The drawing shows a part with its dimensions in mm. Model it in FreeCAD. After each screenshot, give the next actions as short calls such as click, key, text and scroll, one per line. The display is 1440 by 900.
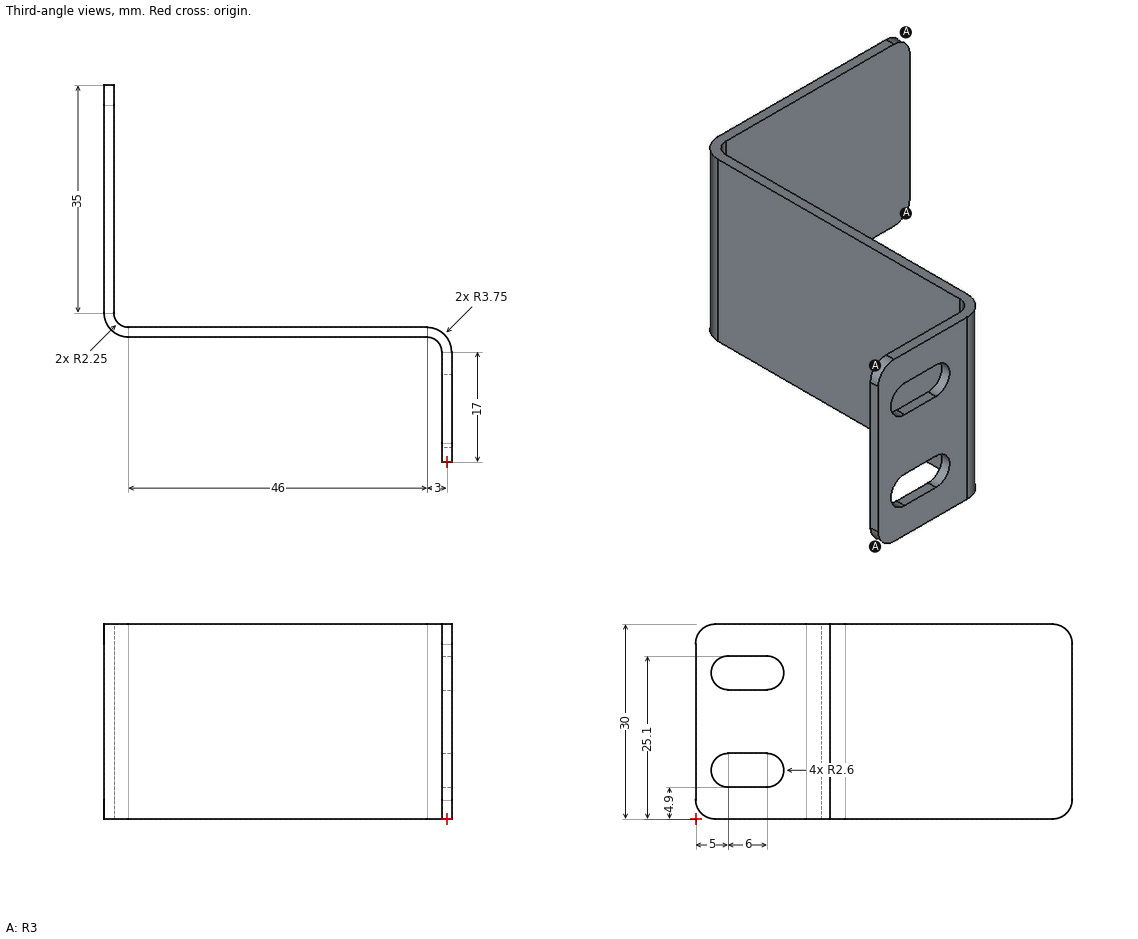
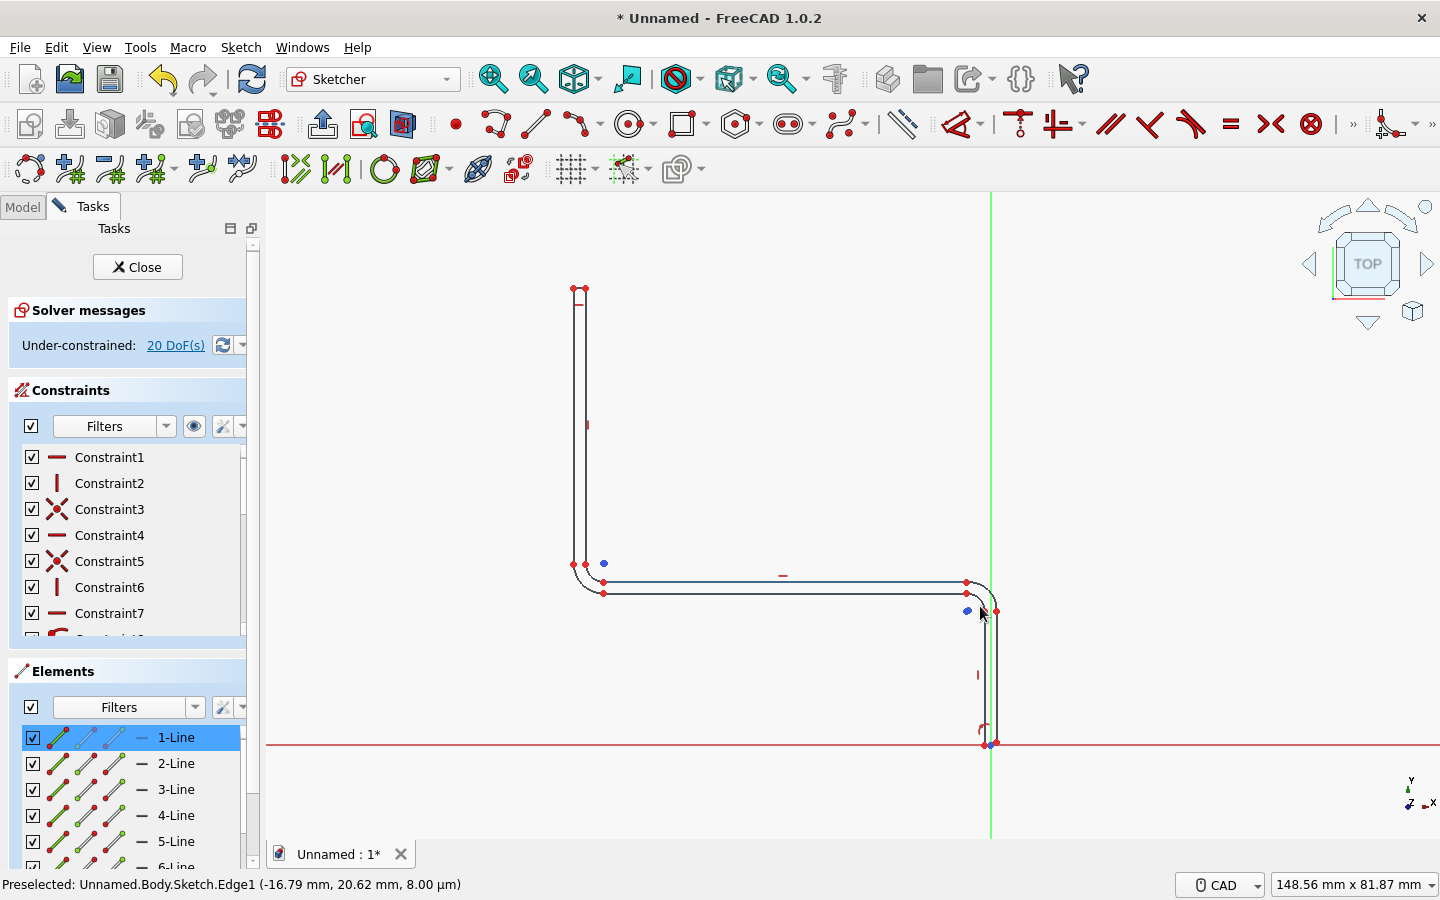
scroll(588, 572, up, 3)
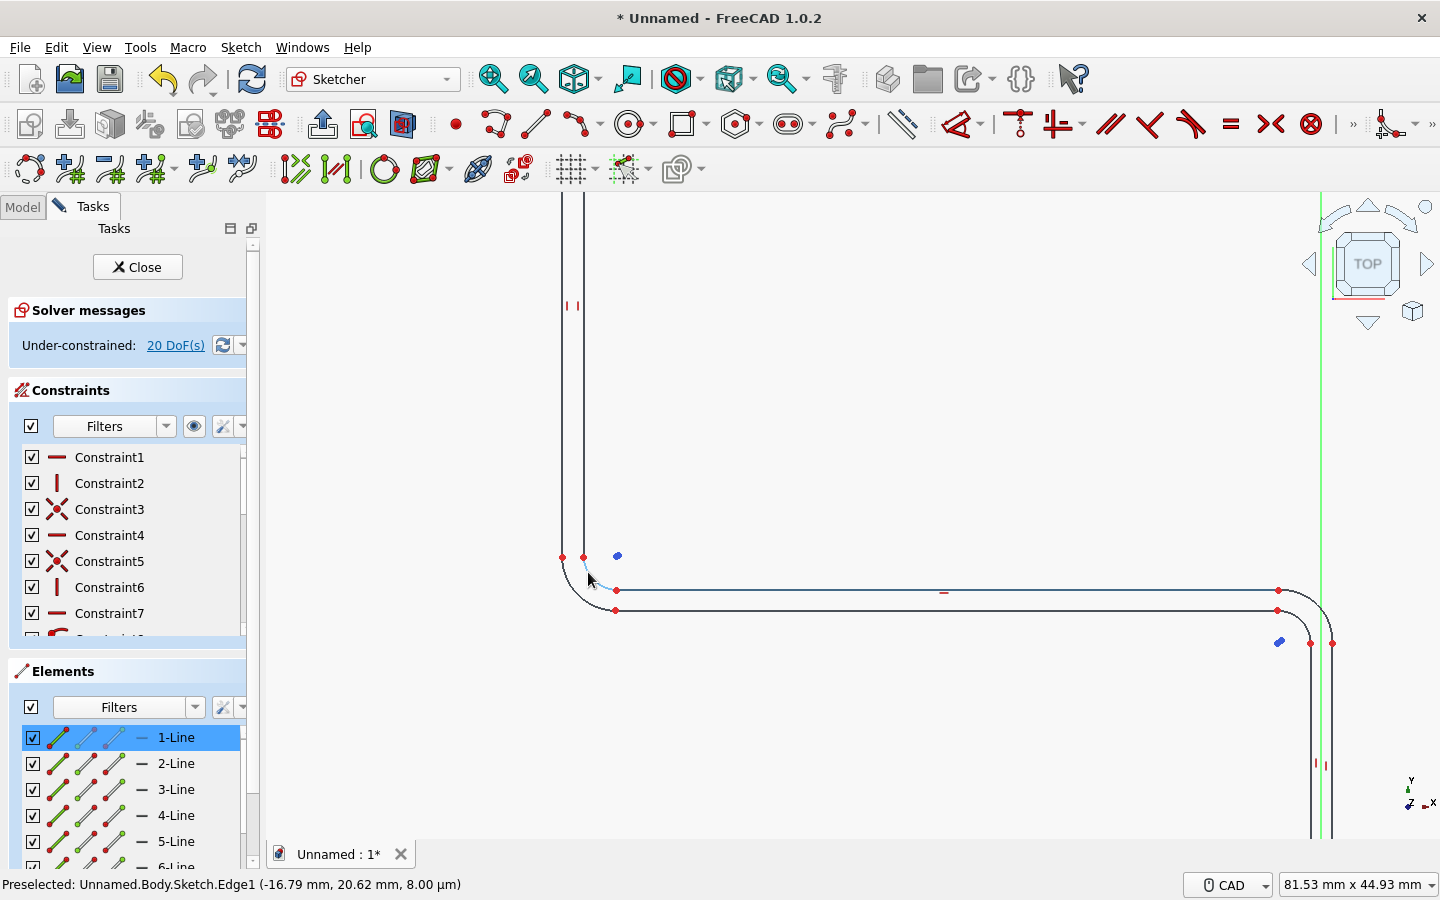
click(588, 572)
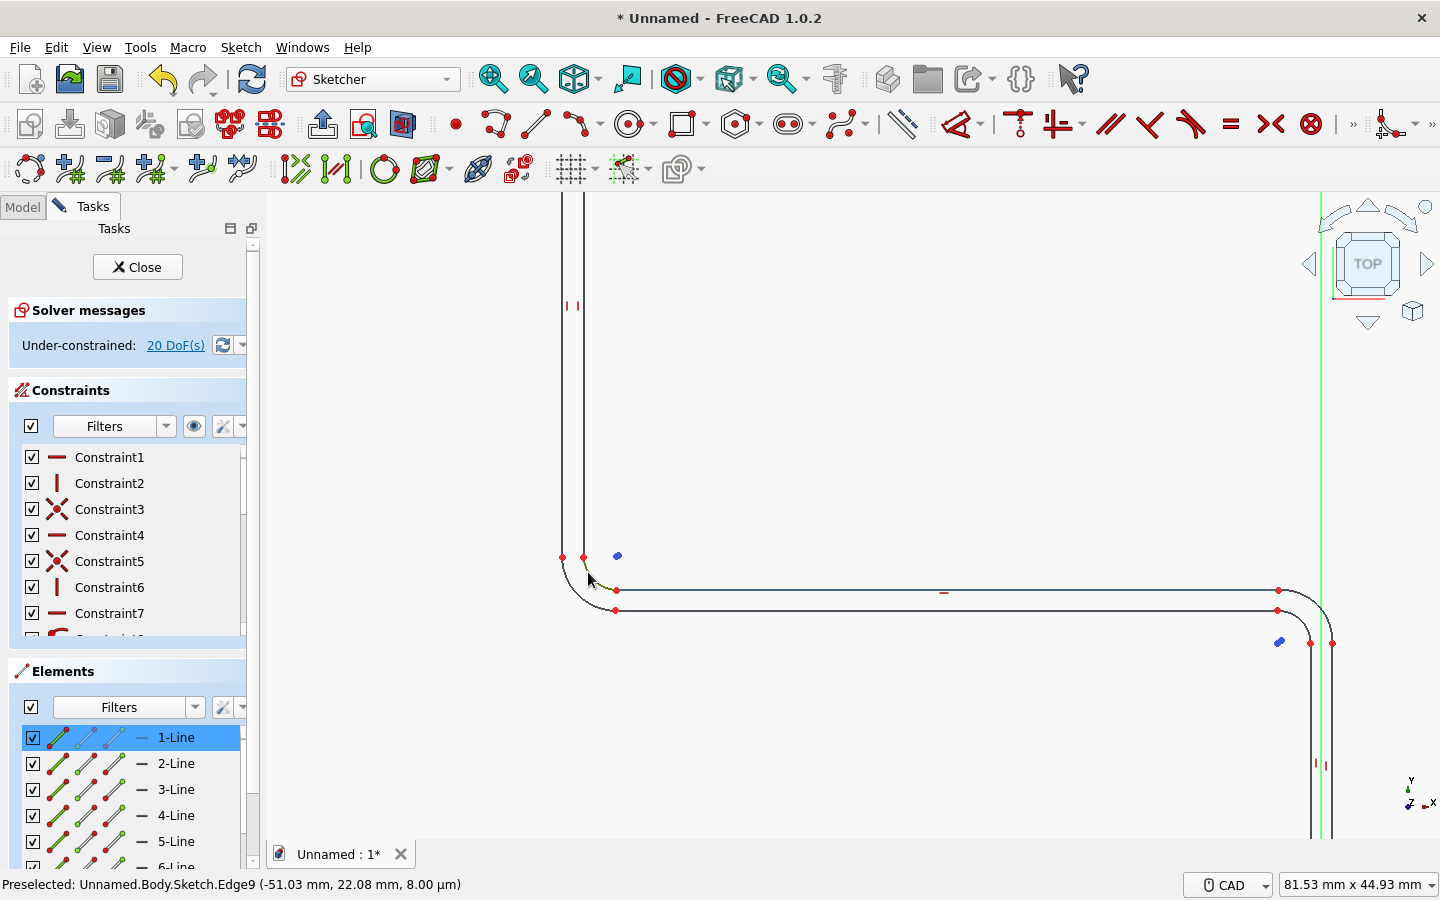
key(t)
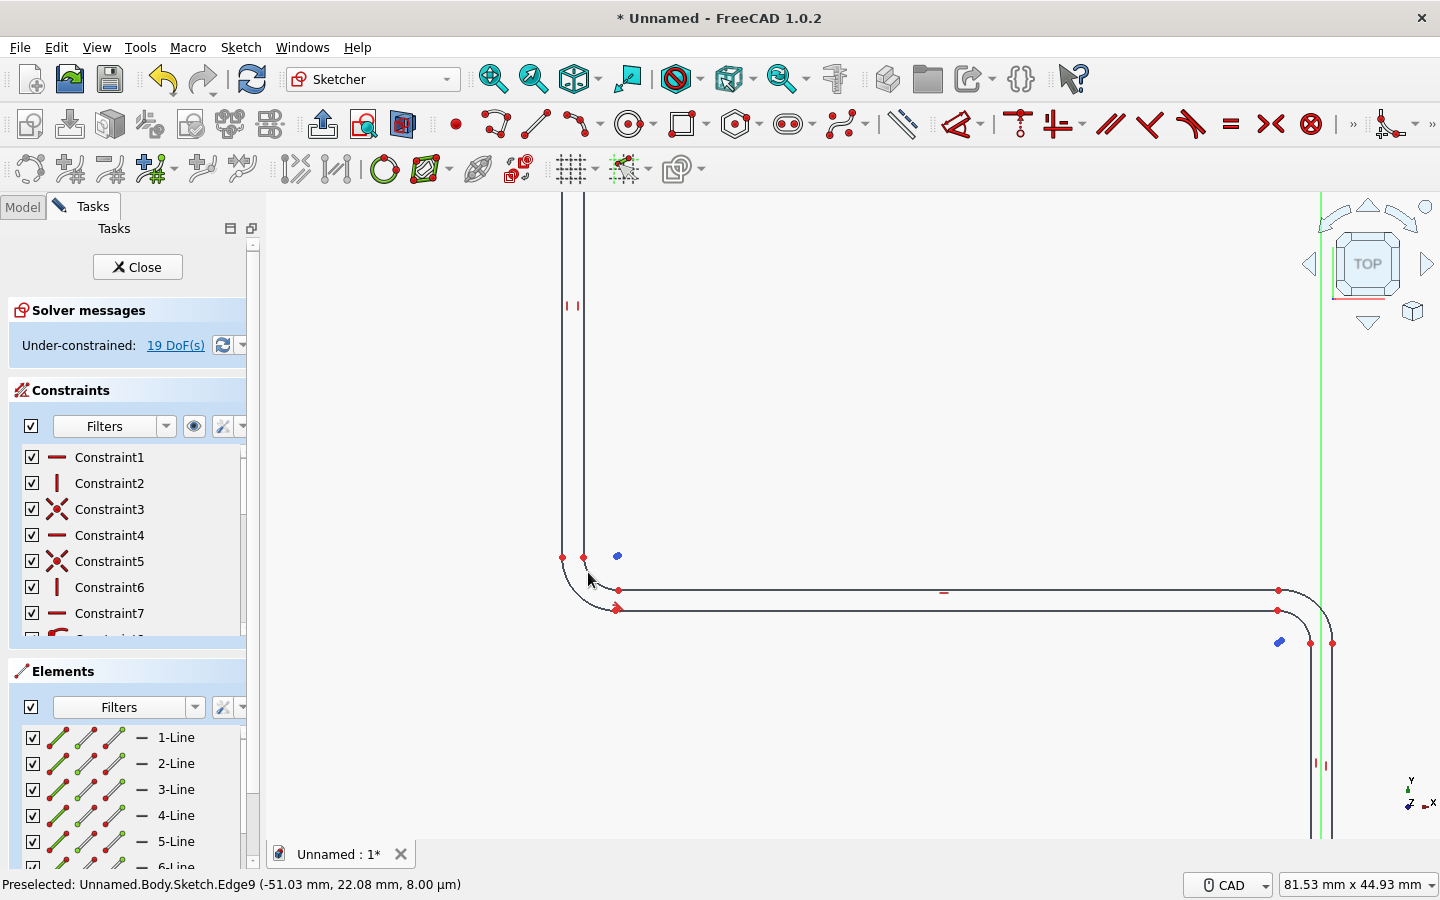
click(1080, 590)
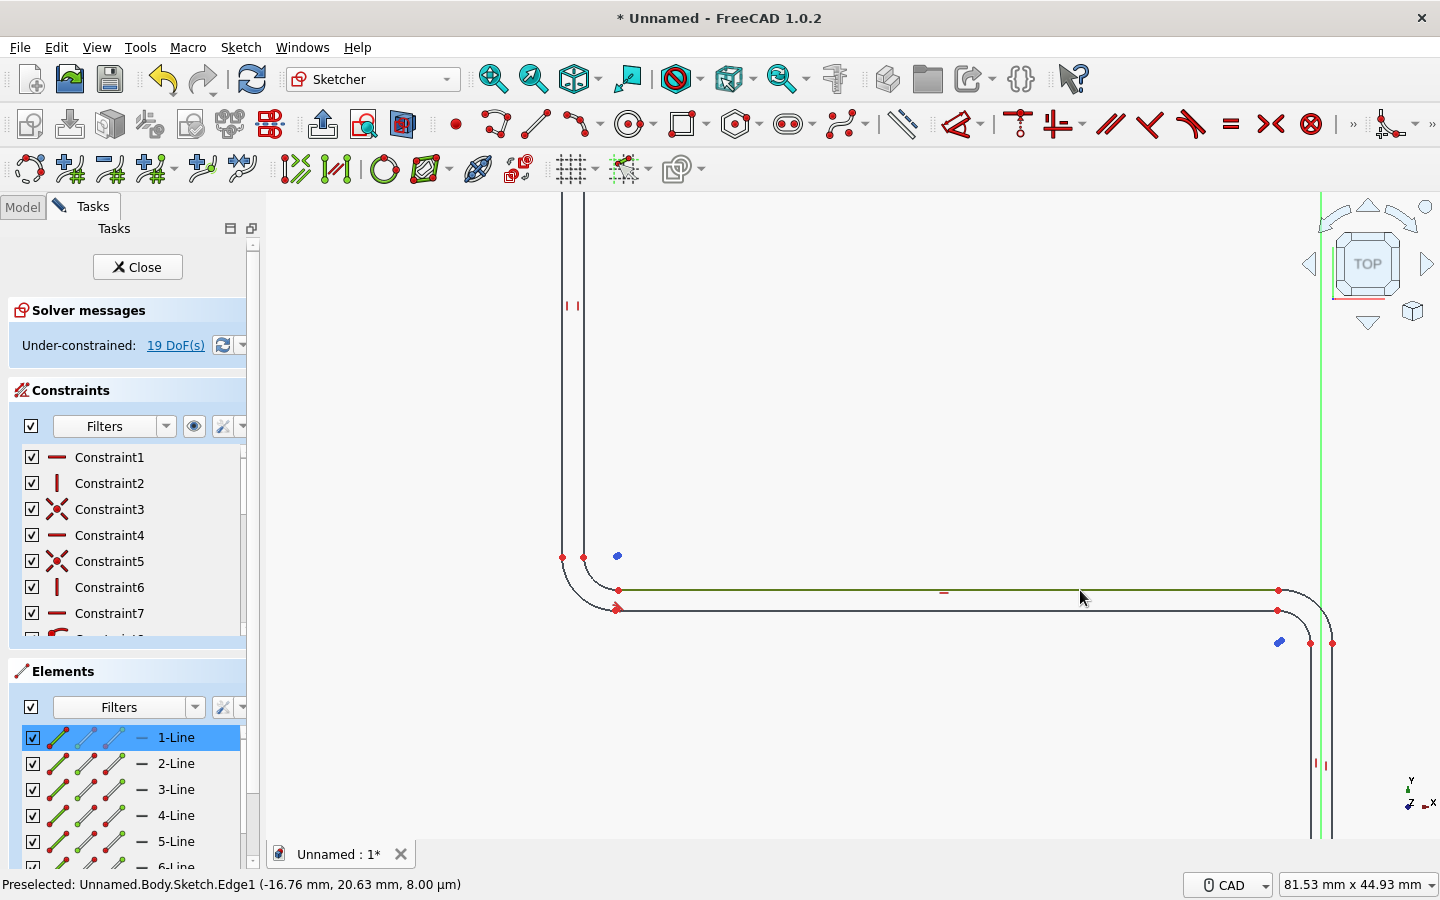
scroll(587, 571, down, 3)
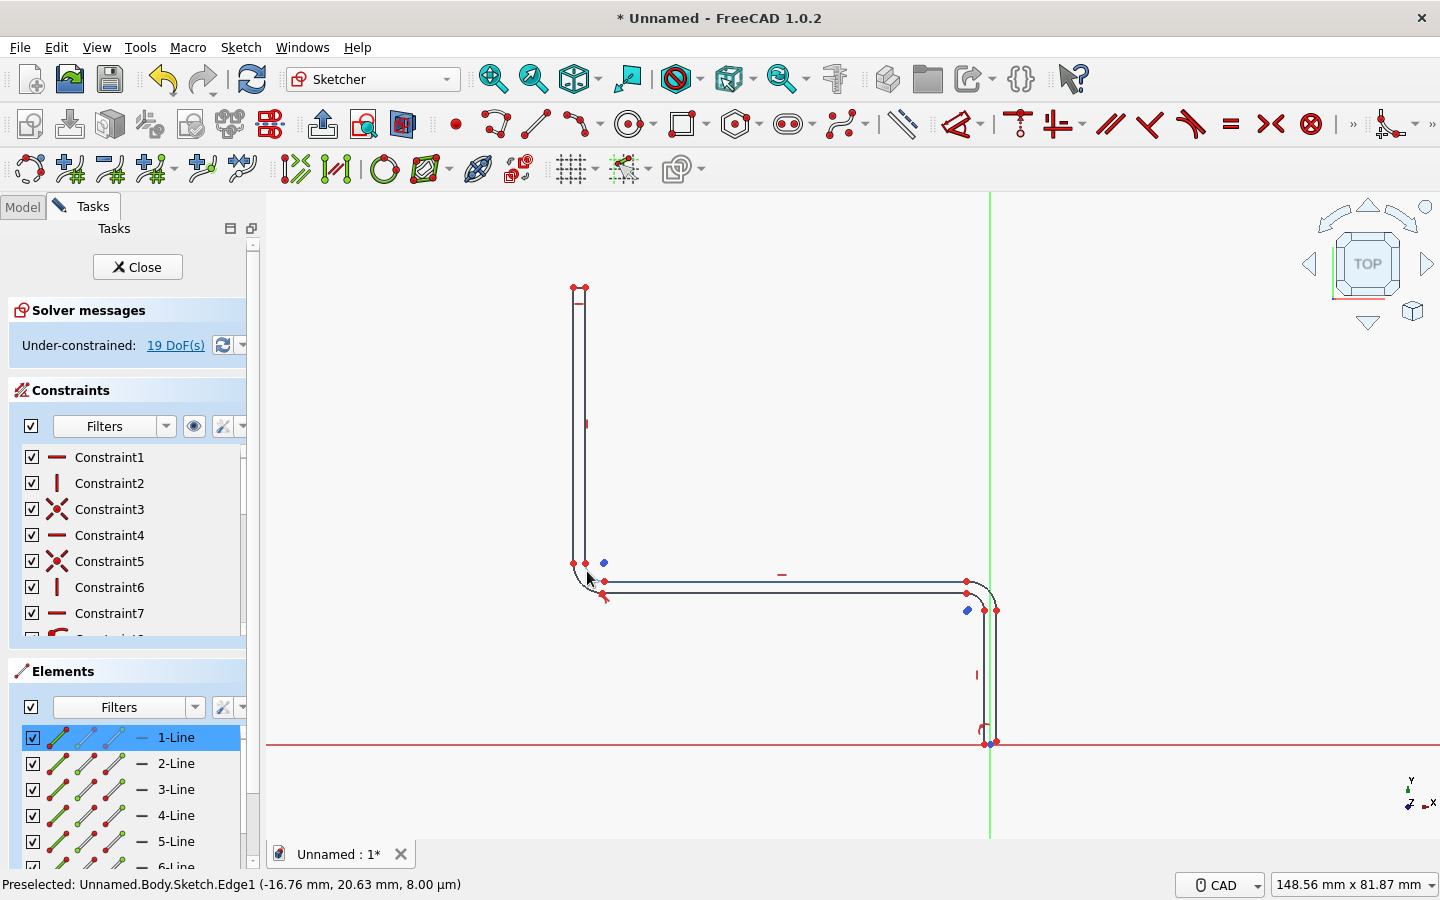
scroll(980, 584, up, 2)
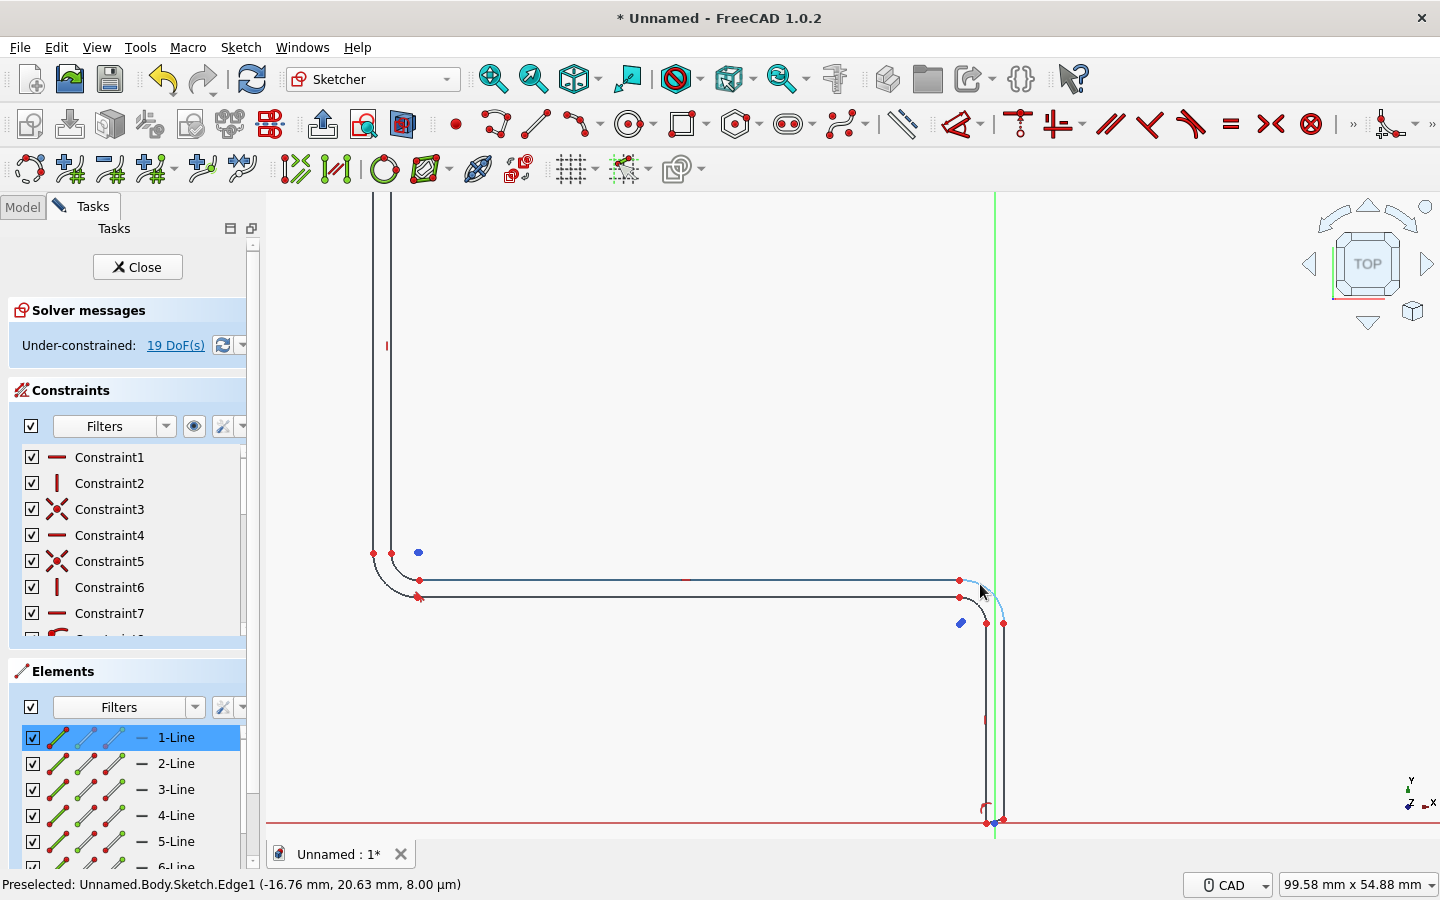
click(980, 584)